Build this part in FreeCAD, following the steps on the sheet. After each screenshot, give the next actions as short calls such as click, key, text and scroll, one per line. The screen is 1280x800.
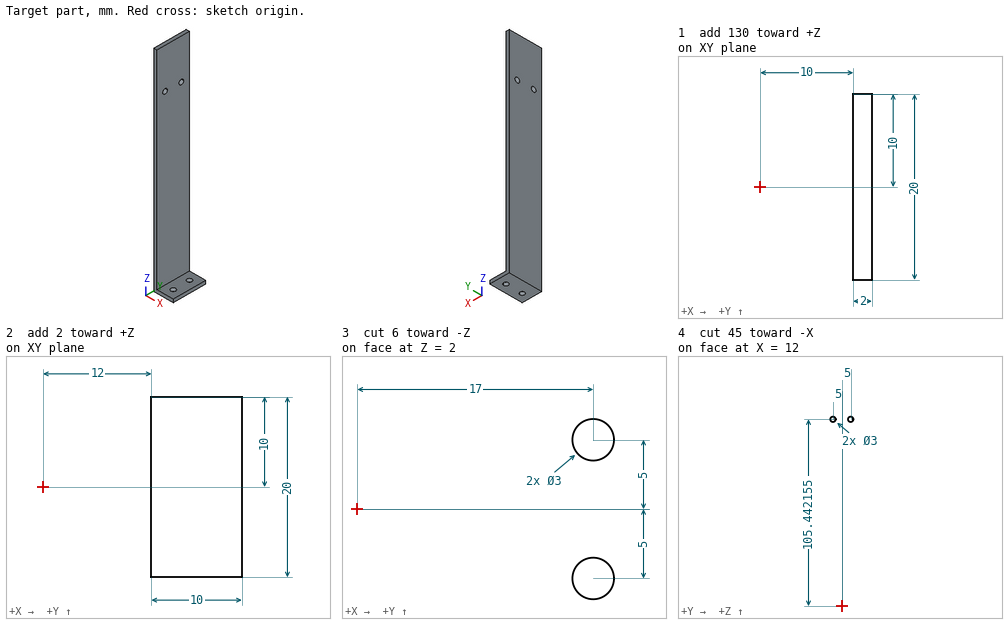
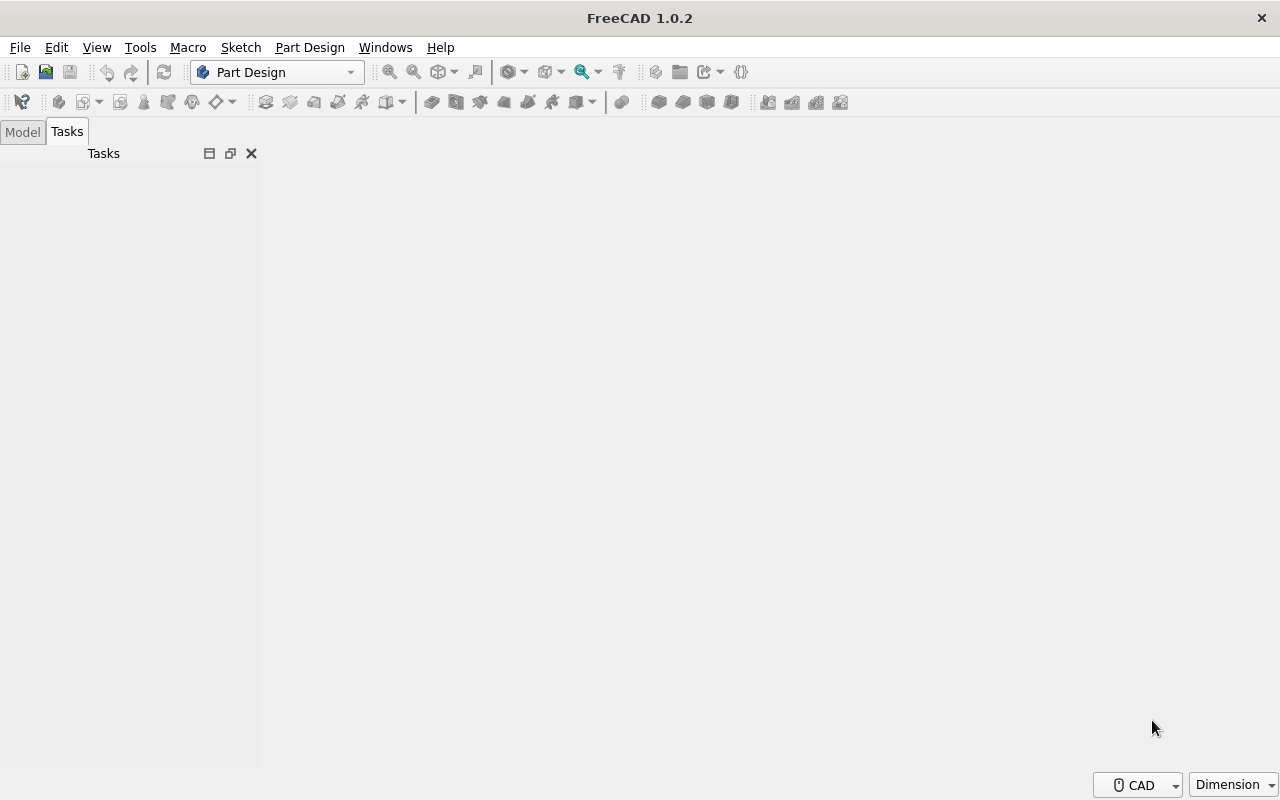
key(ctrl+n)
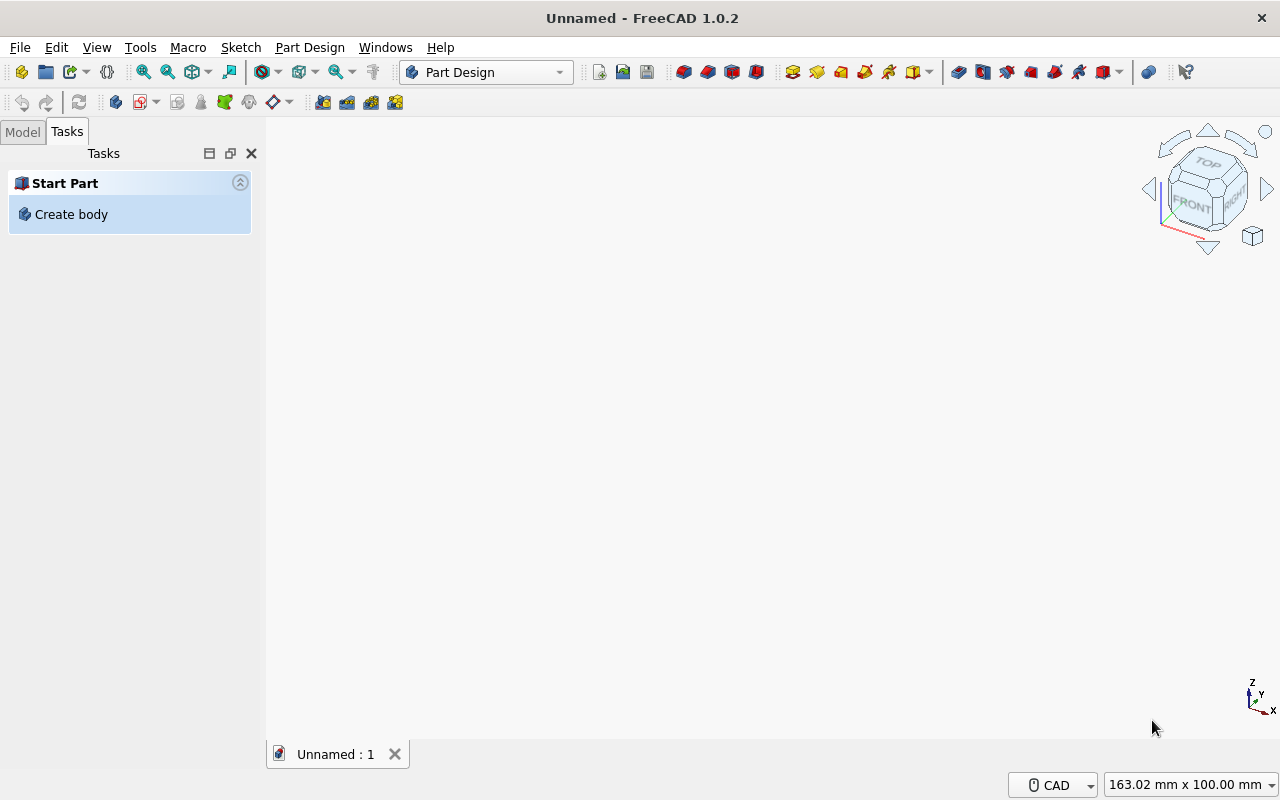
click(140, 102)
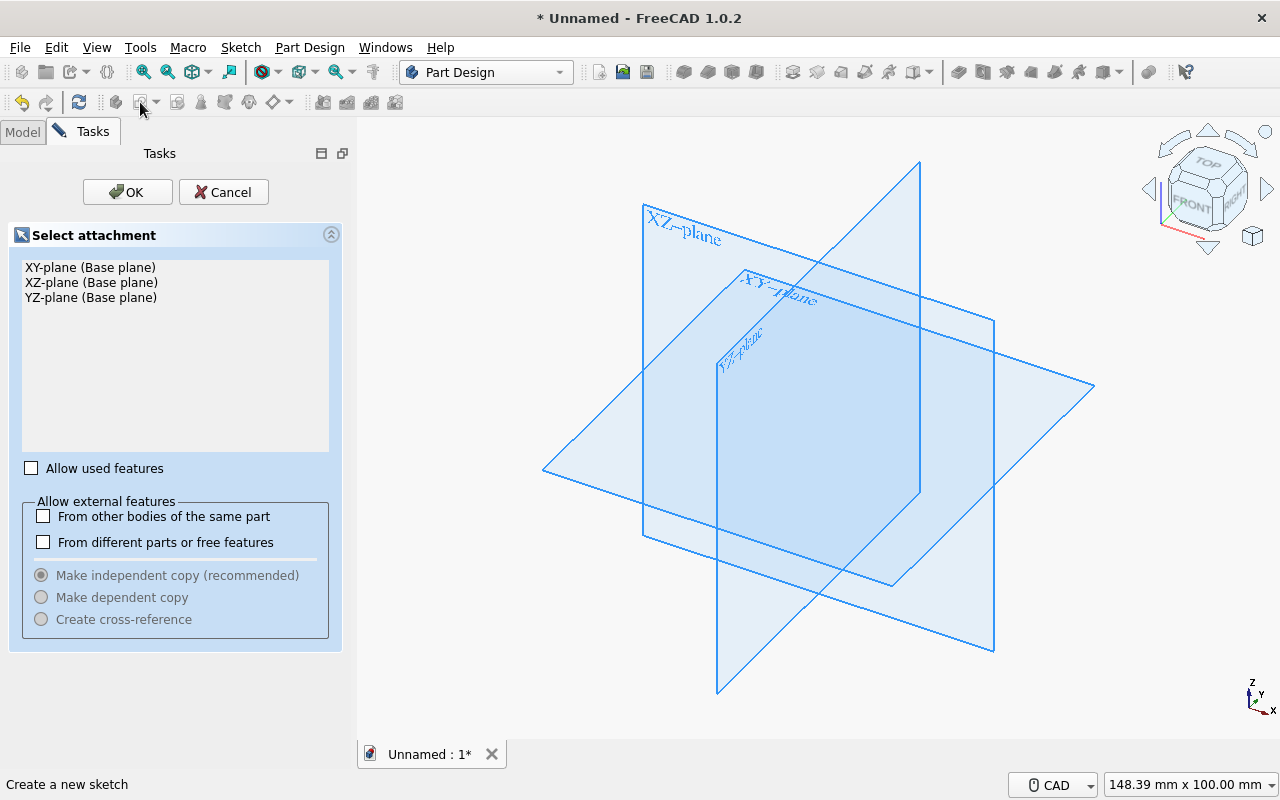
click(82, 268)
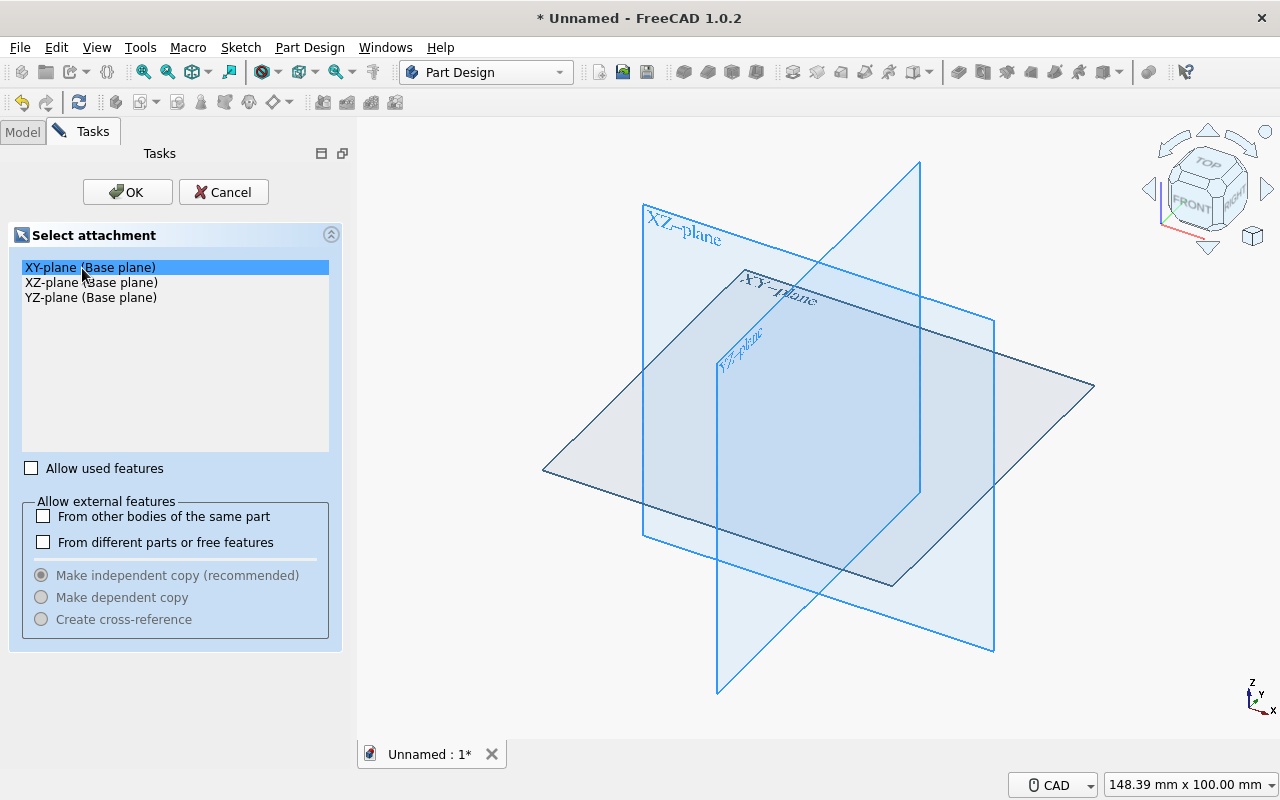
click(128, 192)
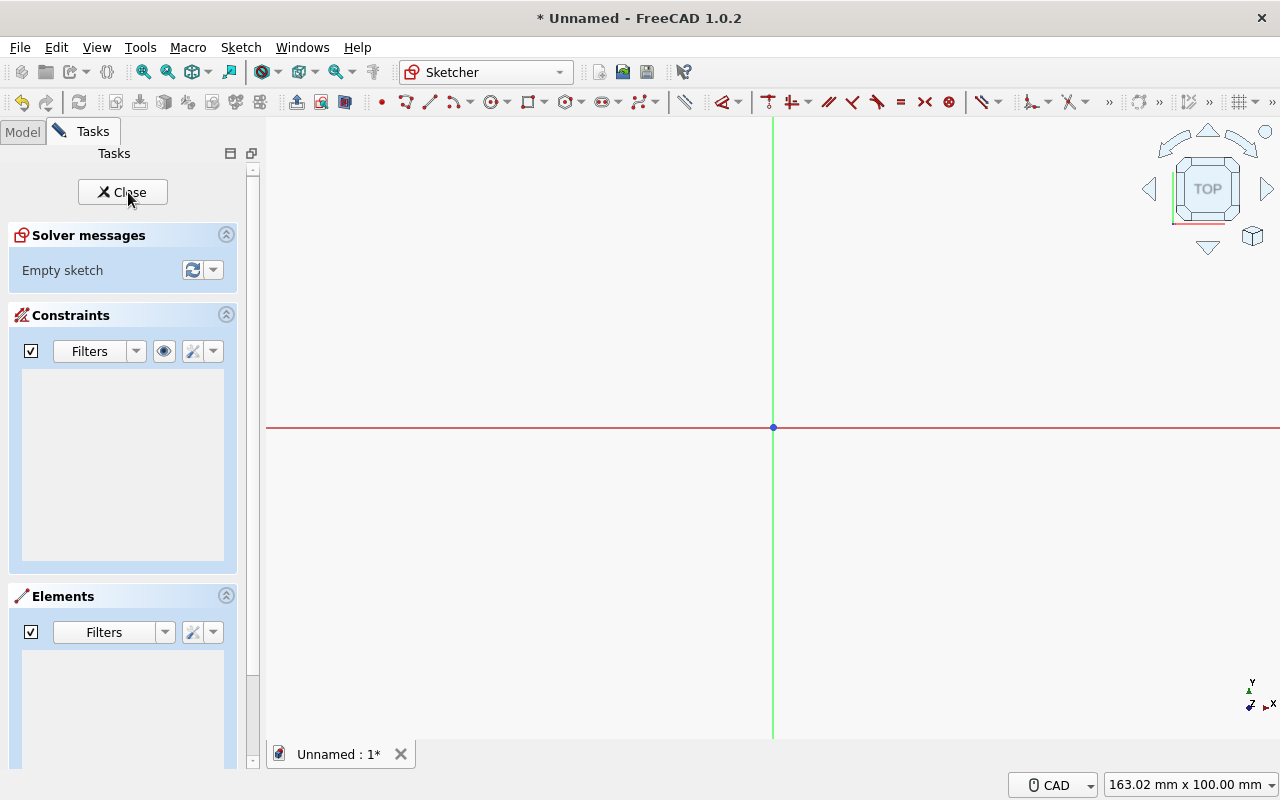
scroll(856, 428, up, 6)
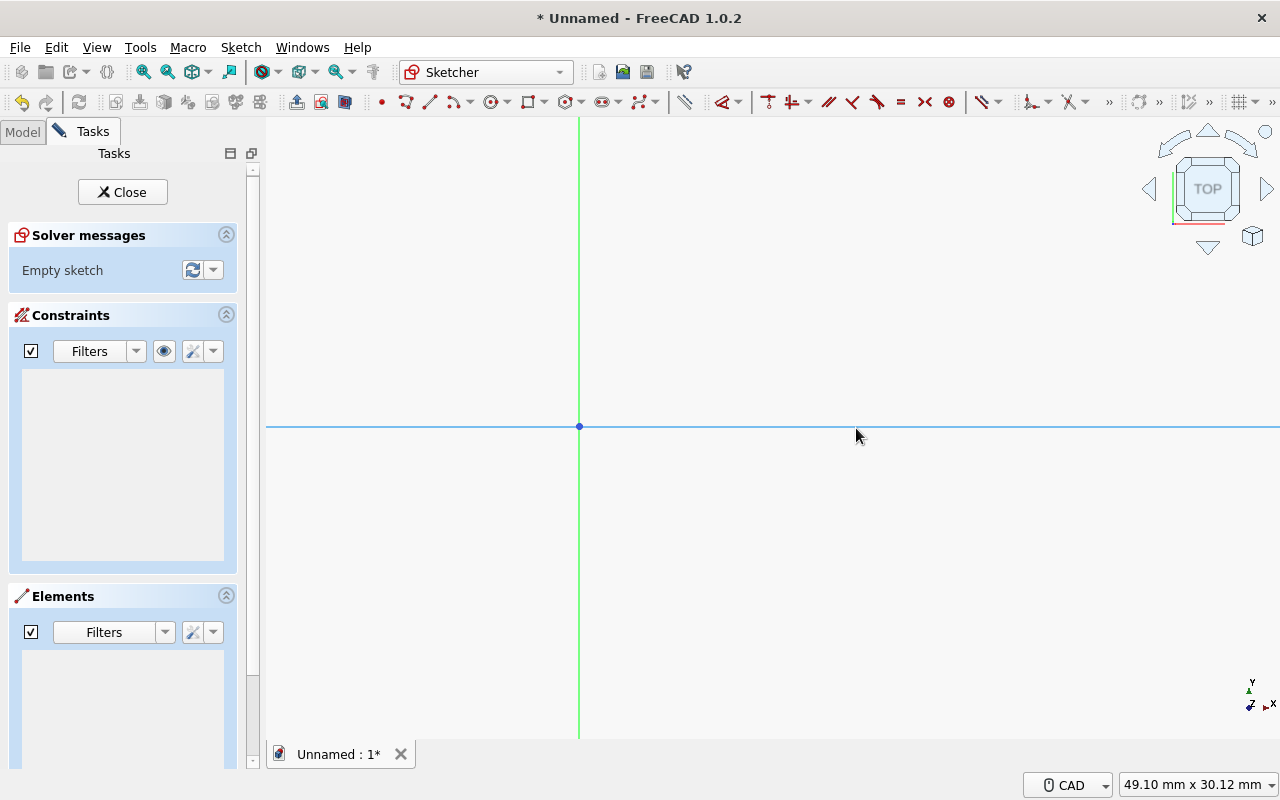
click(528, 102)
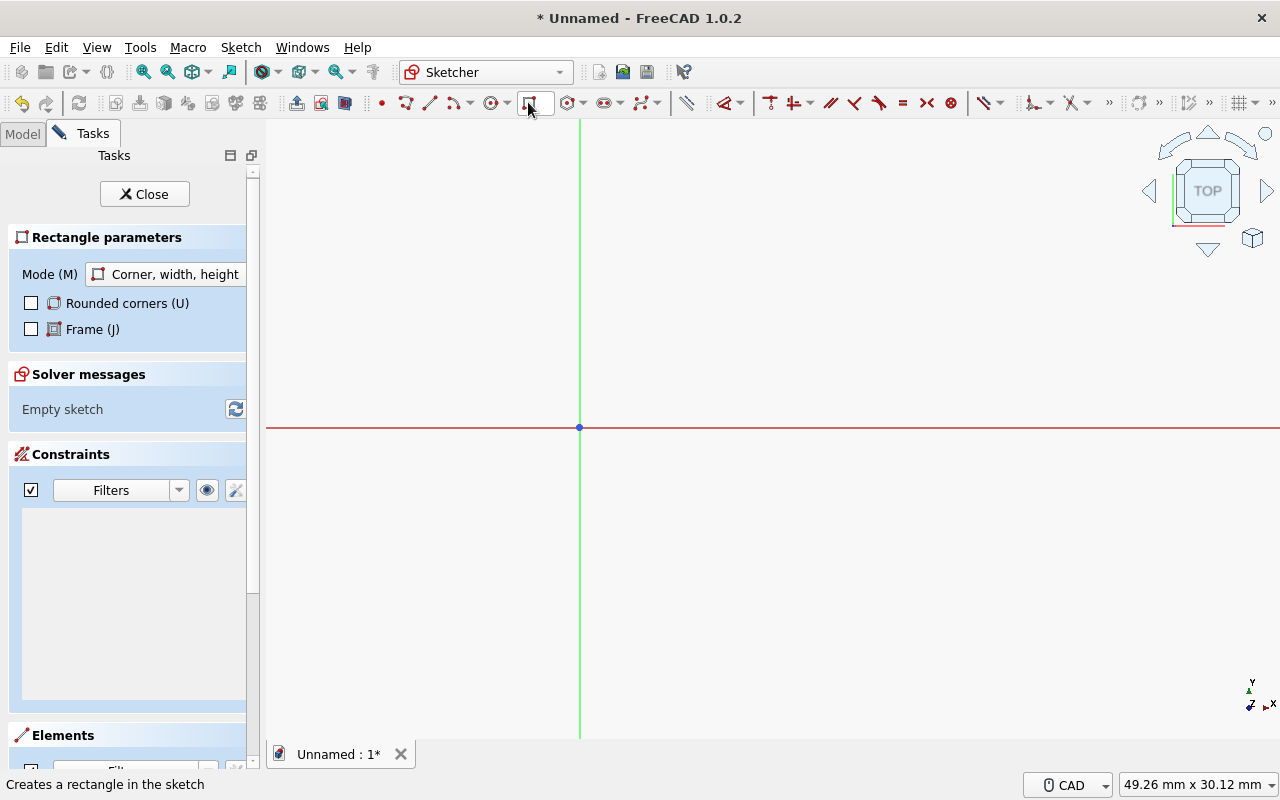
click(786, 222)
move(827, 634)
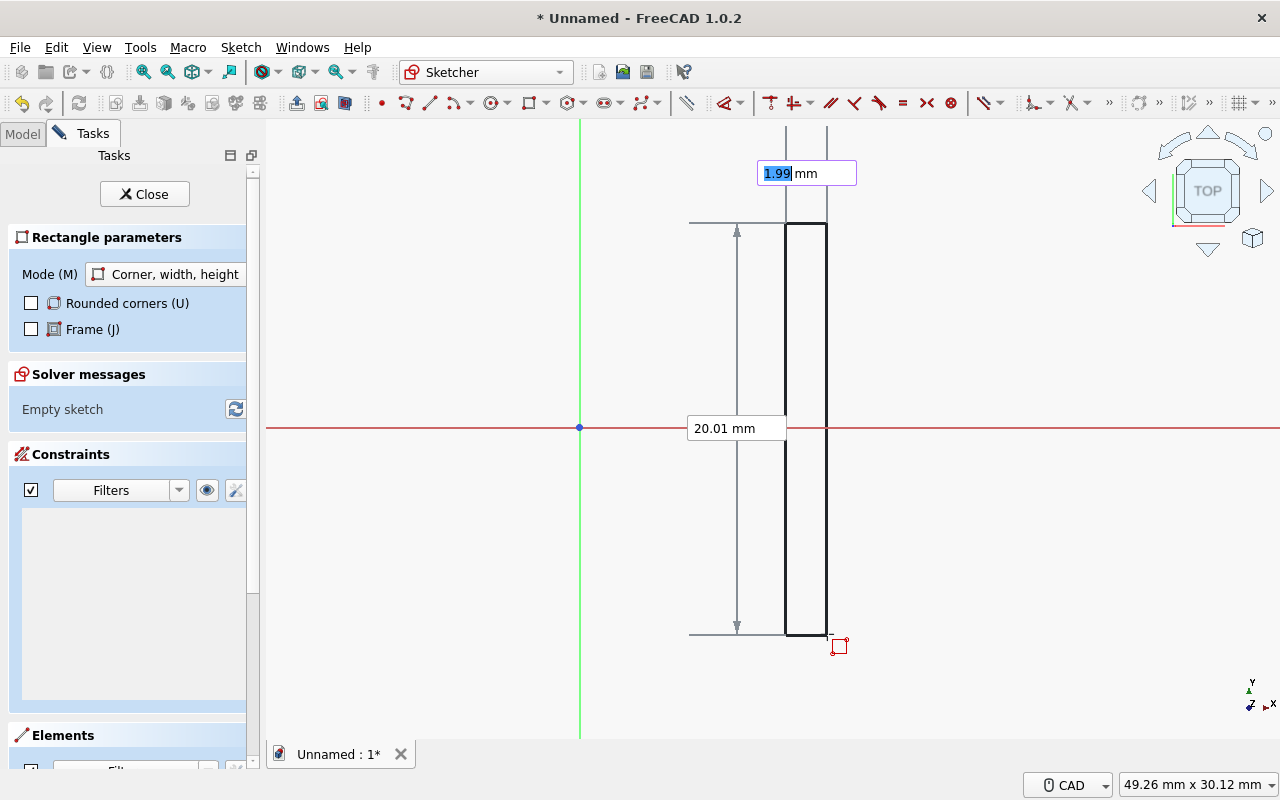
text(2)
key(Tab)
text(20)
key(Return)
key(Escape)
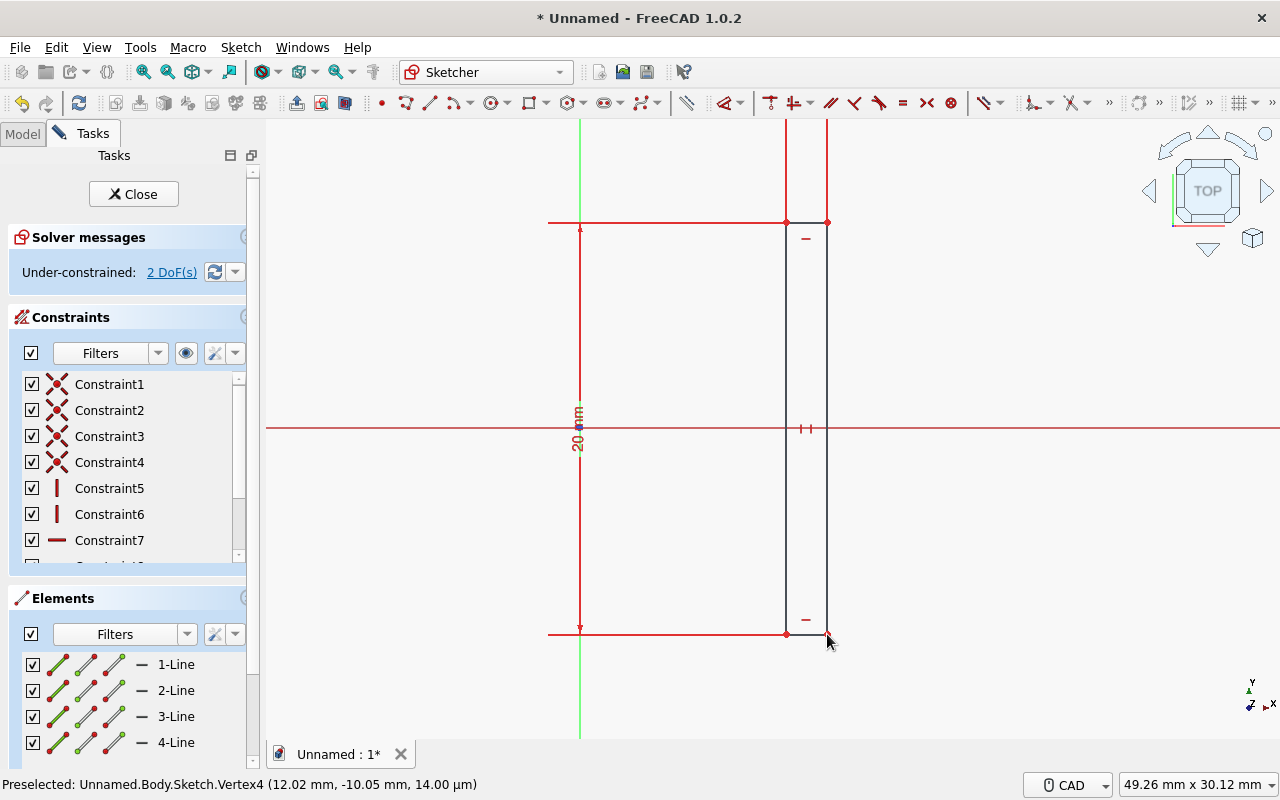
key(d)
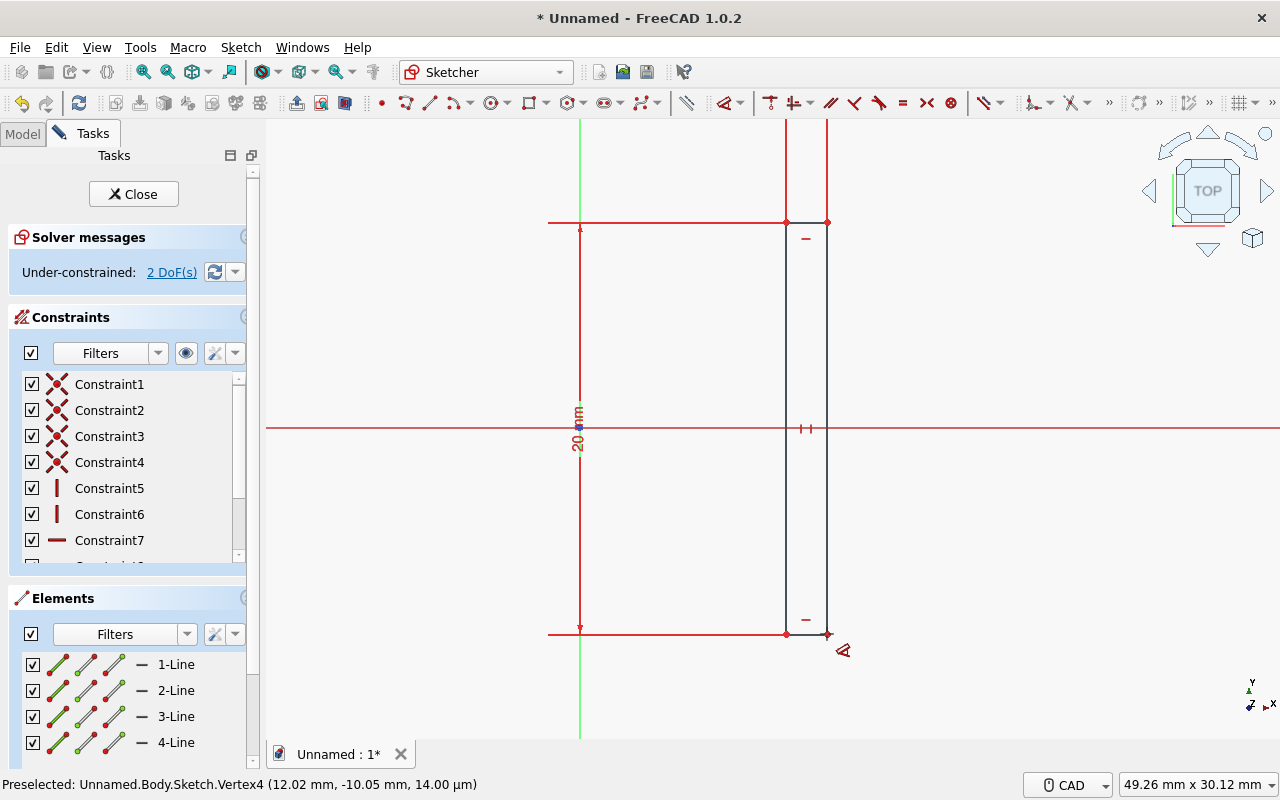
click(786, 223)
click(683, 189)